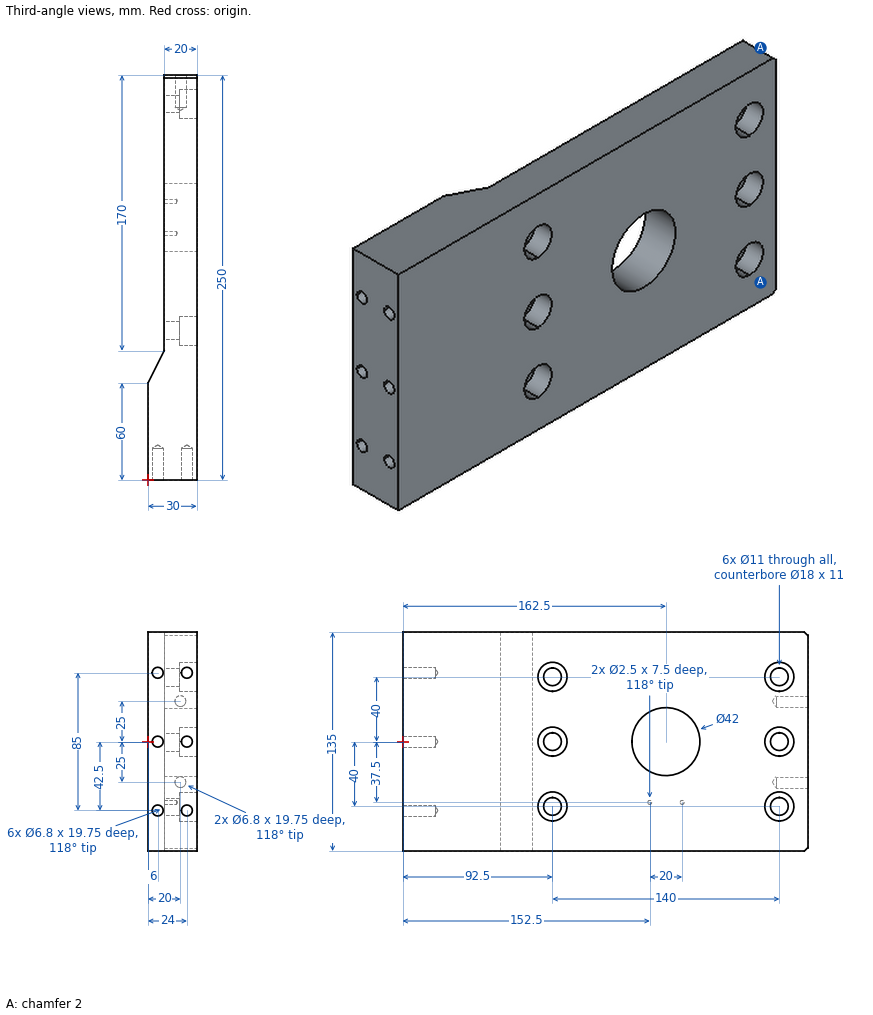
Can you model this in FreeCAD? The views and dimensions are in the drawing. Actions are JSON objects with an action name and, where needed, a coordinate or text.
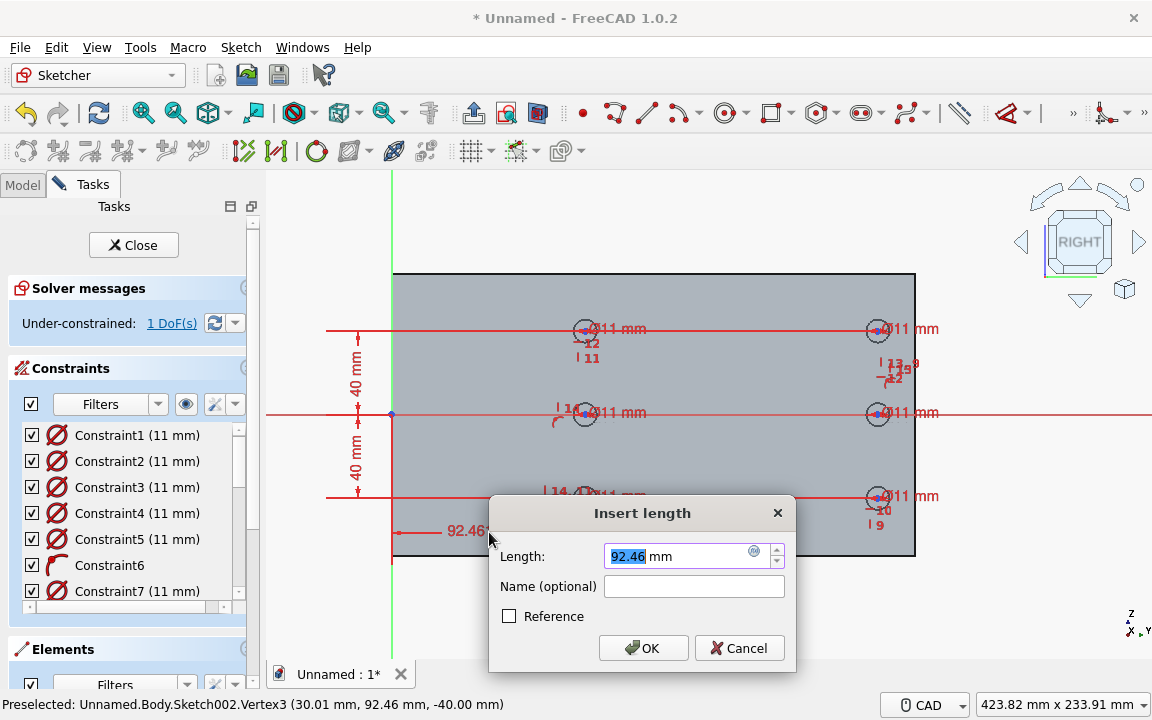
{"action": "type", "text": "92.5"}
{"action": "key", "text": "Return"}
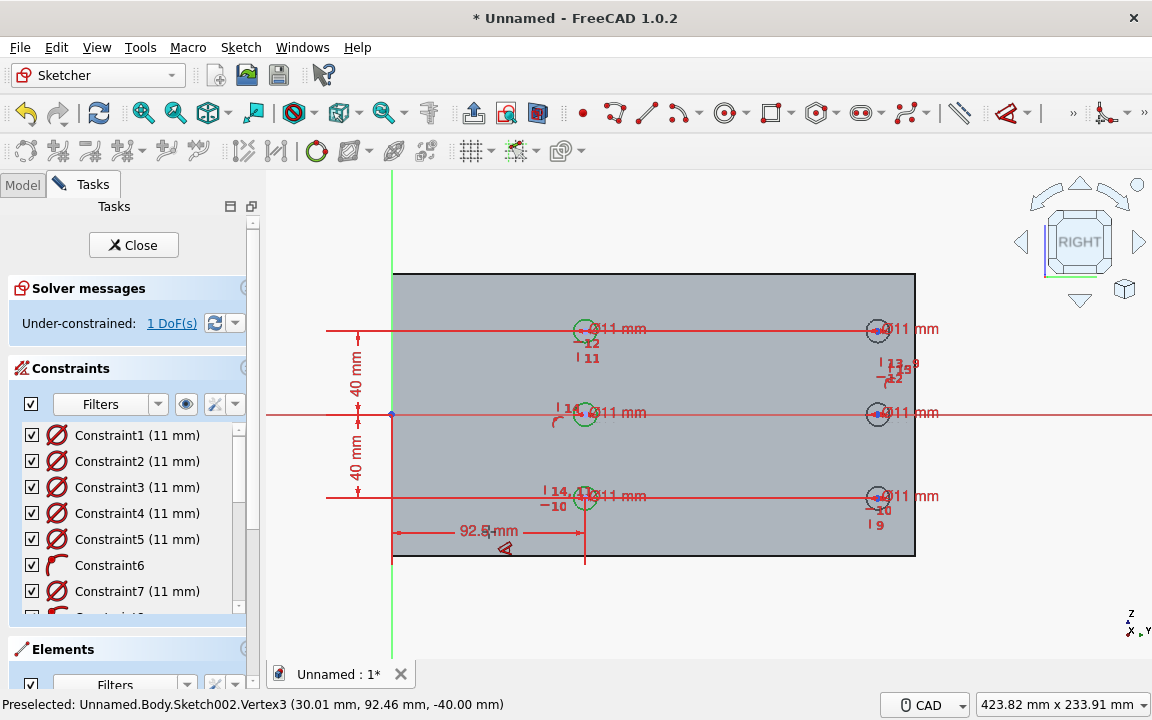
{"action": "left_click", "coordinate": [878, 498]}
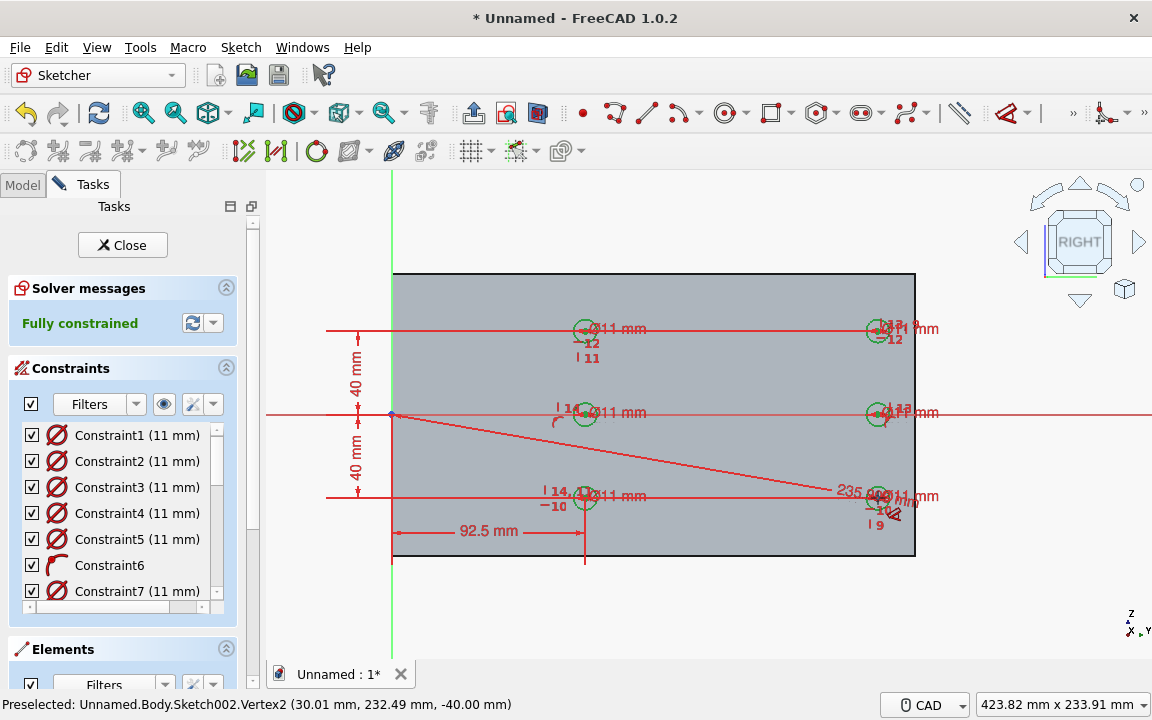
{"action": "left_click", "coordinate": [585, 498]}
{"action": "left_click", "coordinate": [732, 532]}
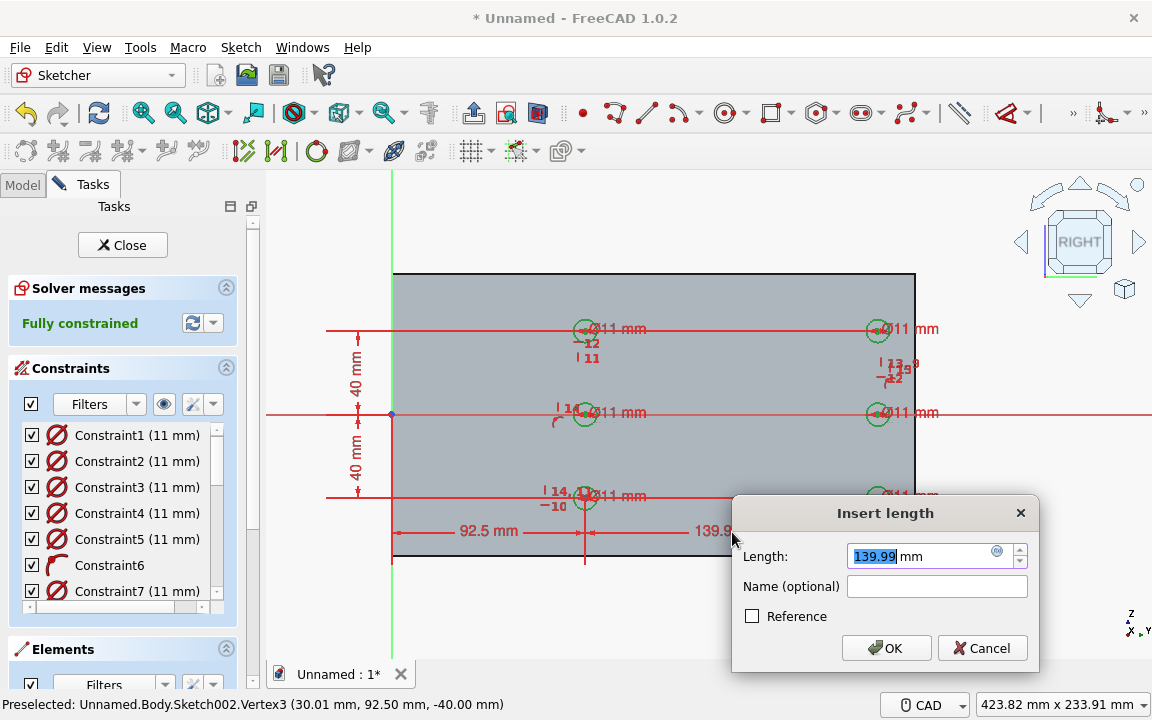
{"action": "type", "text": "140"}
{"action": "key", "text": "Return"}
{"action": "key", "text": "Escape"}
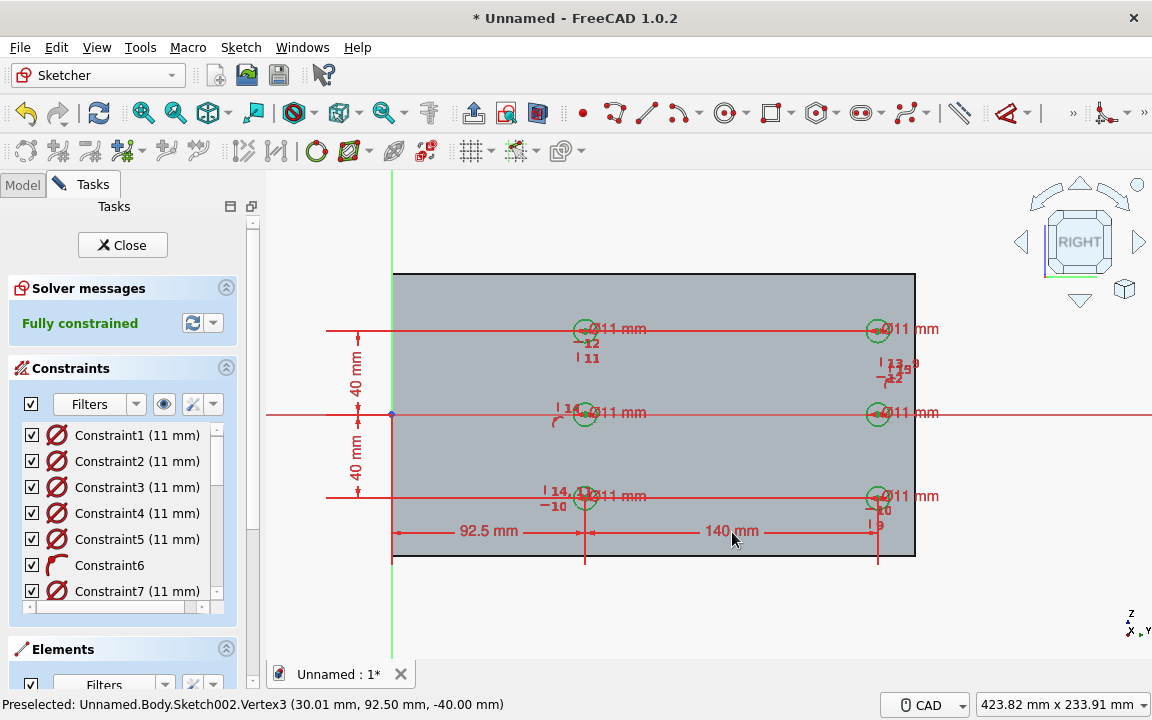
{"action": "left_click", "coordinate": [123, 245]}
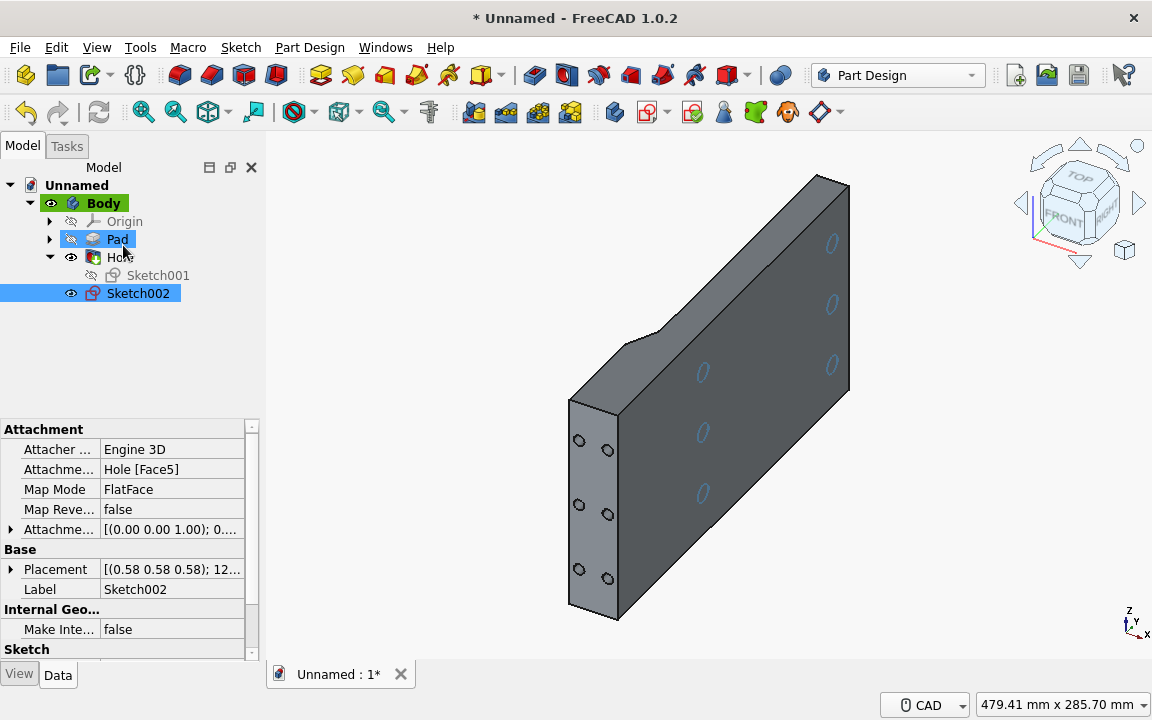
{"action": "left_click", "coordinate": [568, 76]}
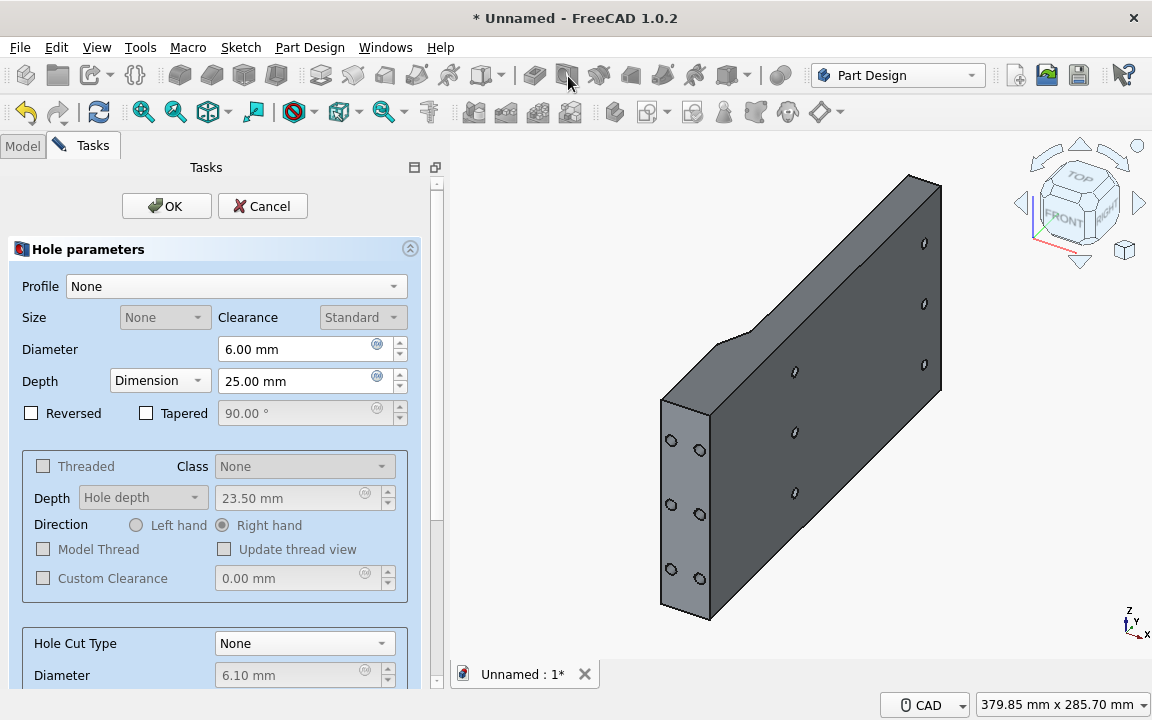
{"action": "triple_click", "coordinate": [305, 349]}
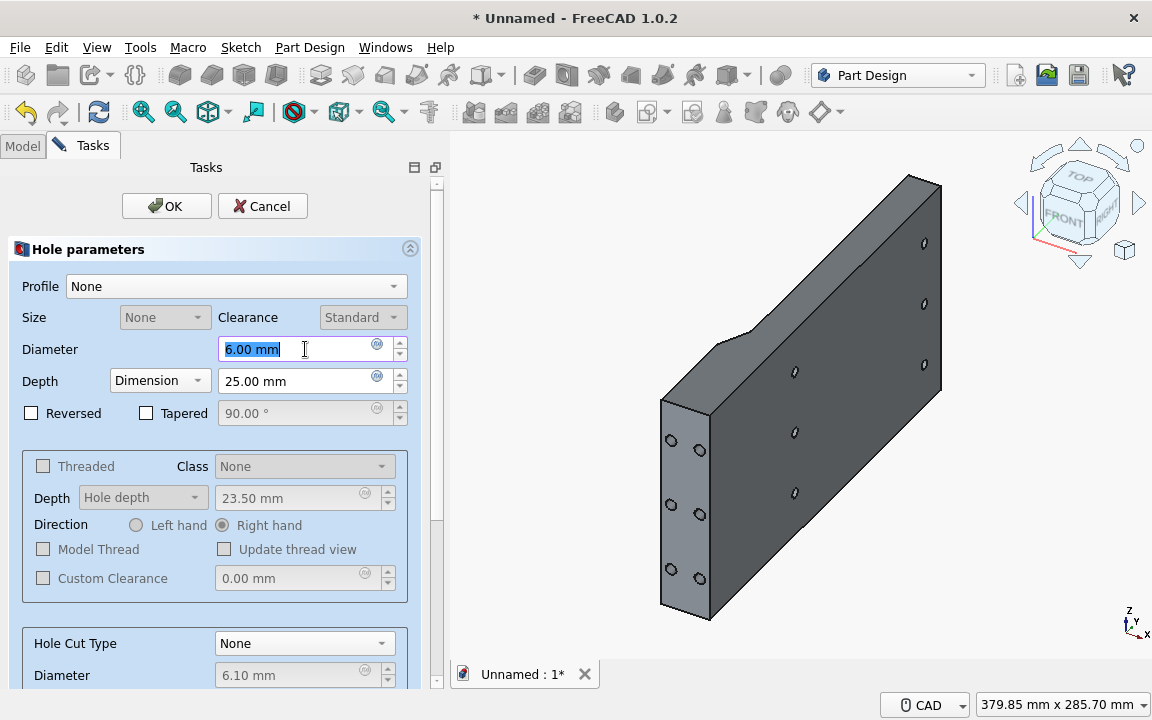
{"action": "type", "text": "11"}
{"action": "key", "text": "Tab"}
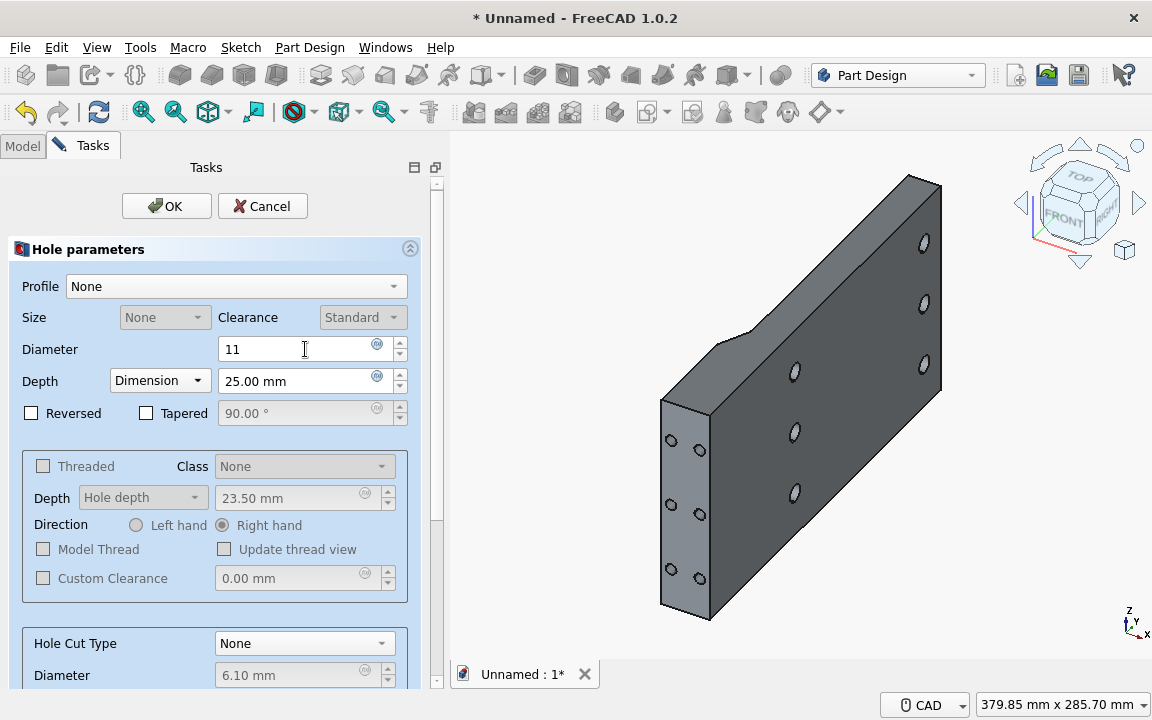
{"action": "left_click", "coordinate": [161, 380]}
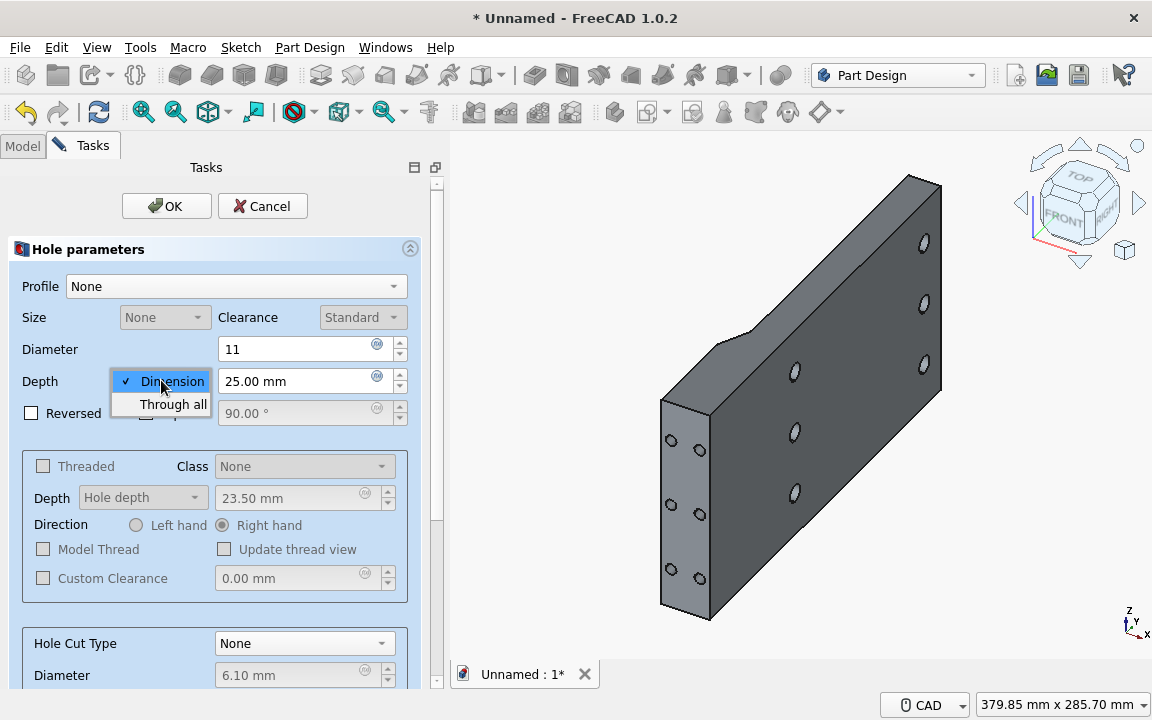
{"action": "left_click", "coordinate": [160, 404]}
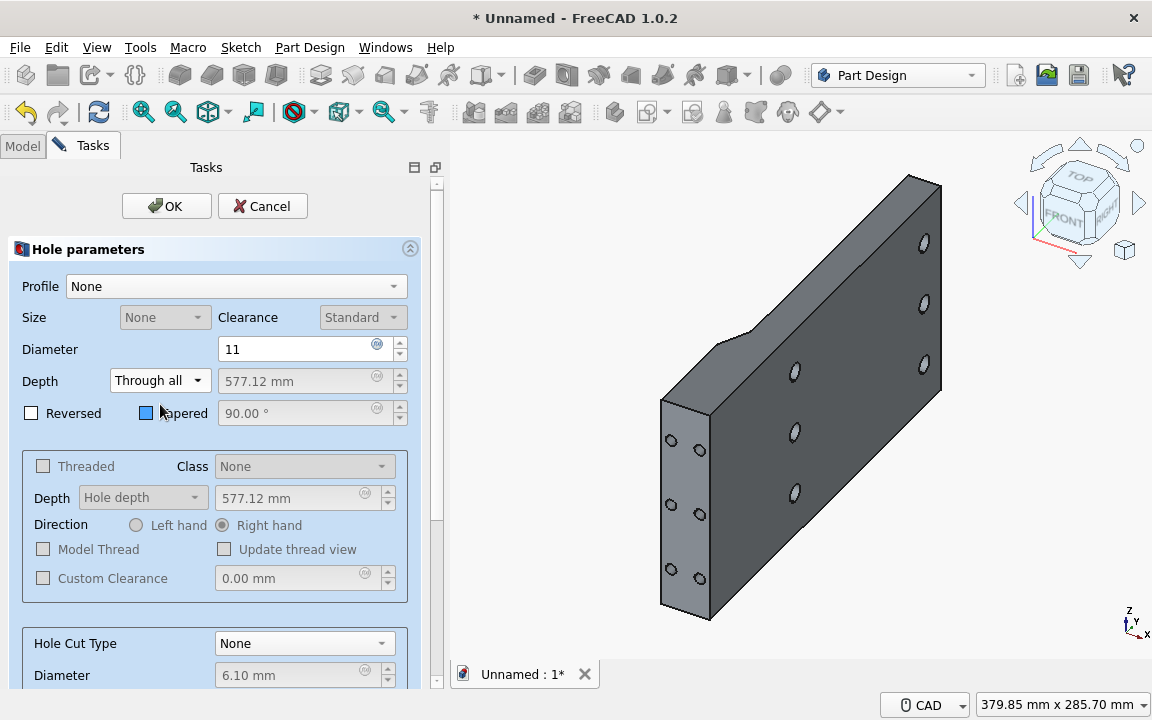
{"action": "left_click", "coordinate": [306, 644]}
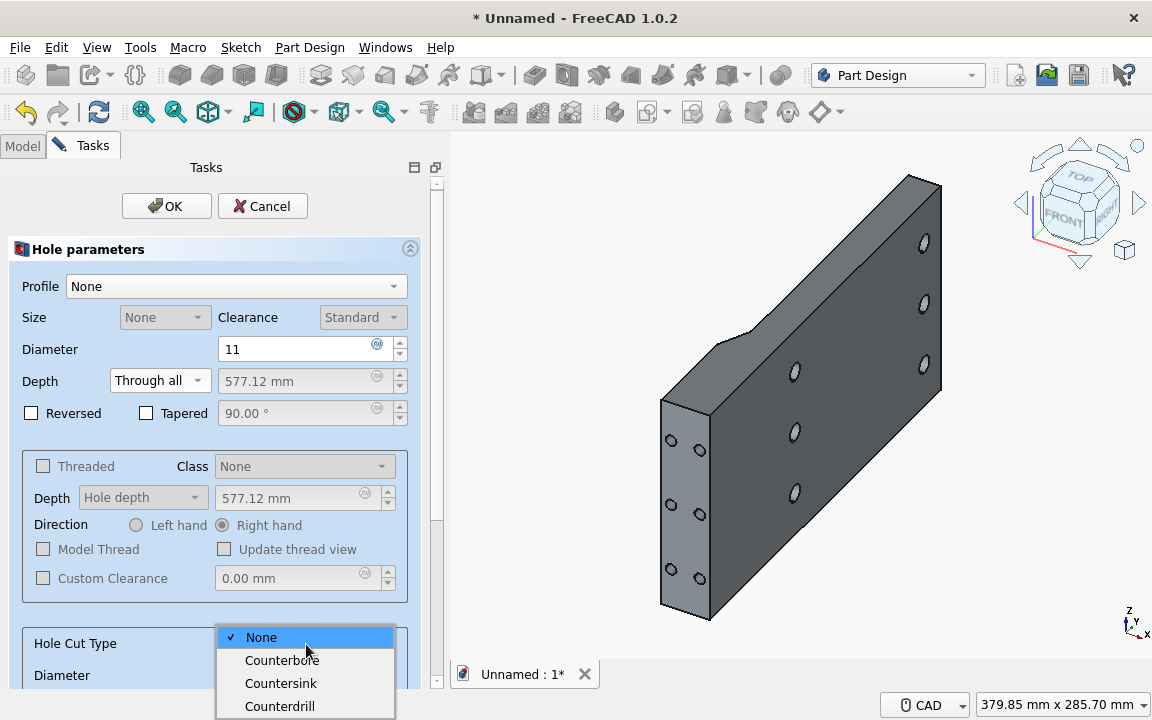
{"action": "left_click", "coordinate": [304, 660]}